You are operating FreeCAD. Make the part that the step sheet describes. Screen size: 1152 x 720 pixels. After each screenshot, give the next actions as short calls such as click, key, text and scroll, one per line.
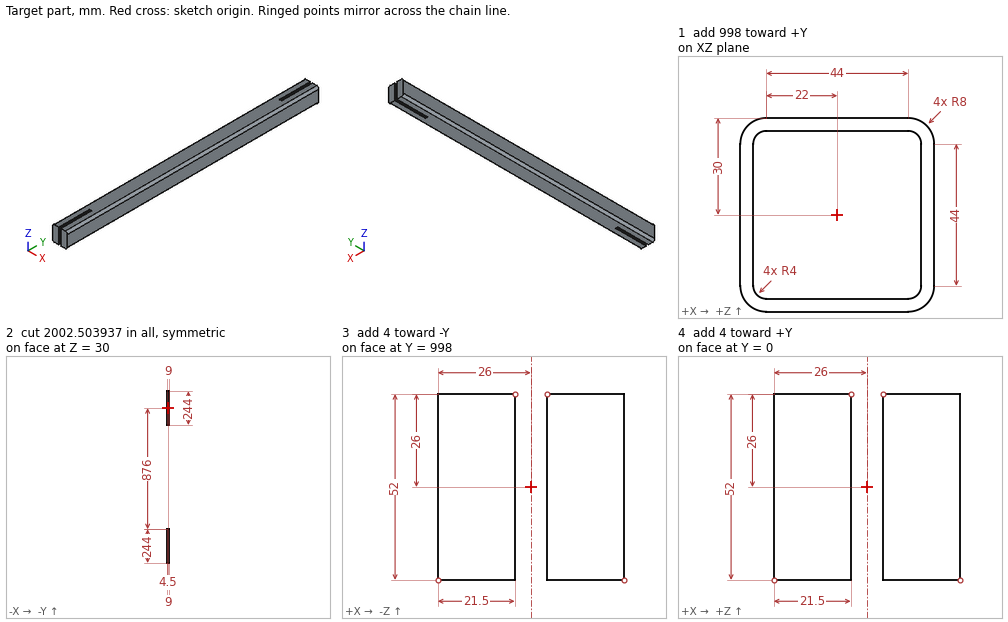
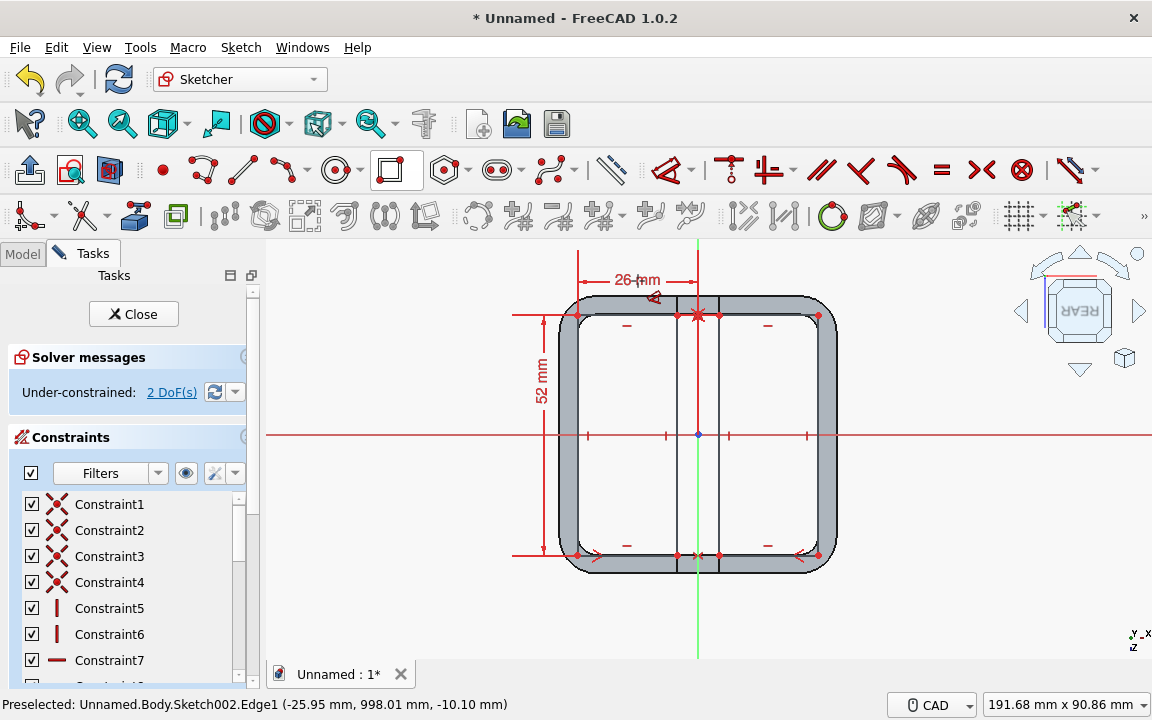
click(578, 315)
click(544, 348)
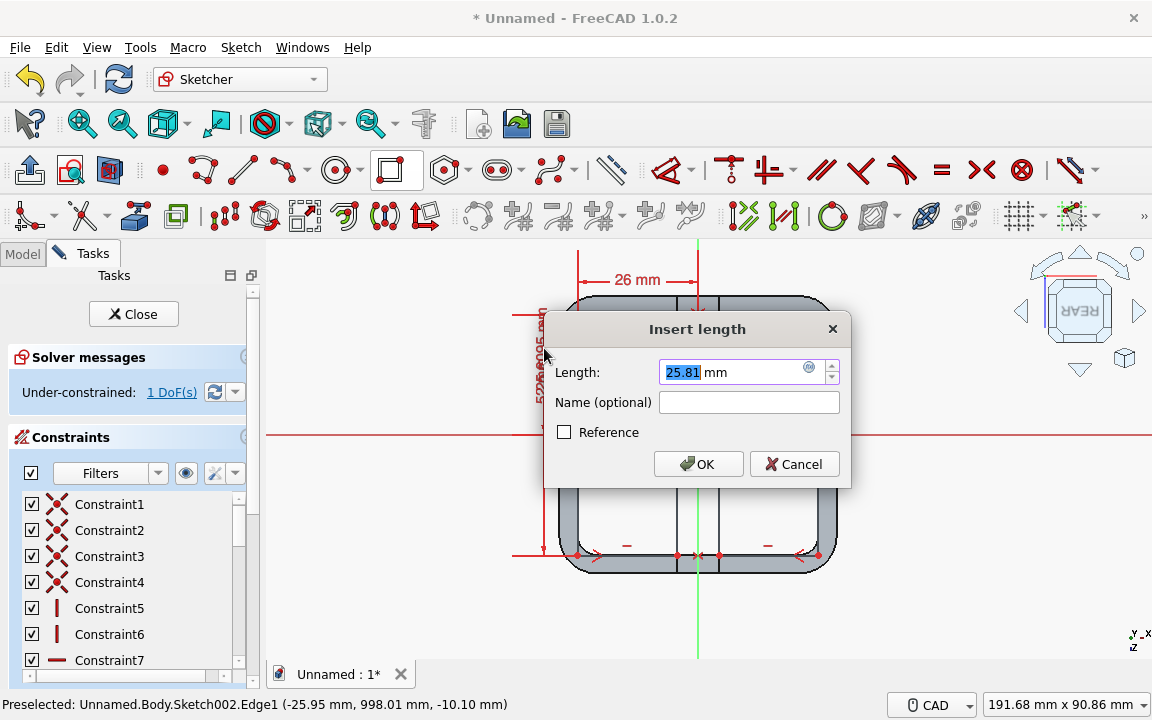
text(26)
key(Return)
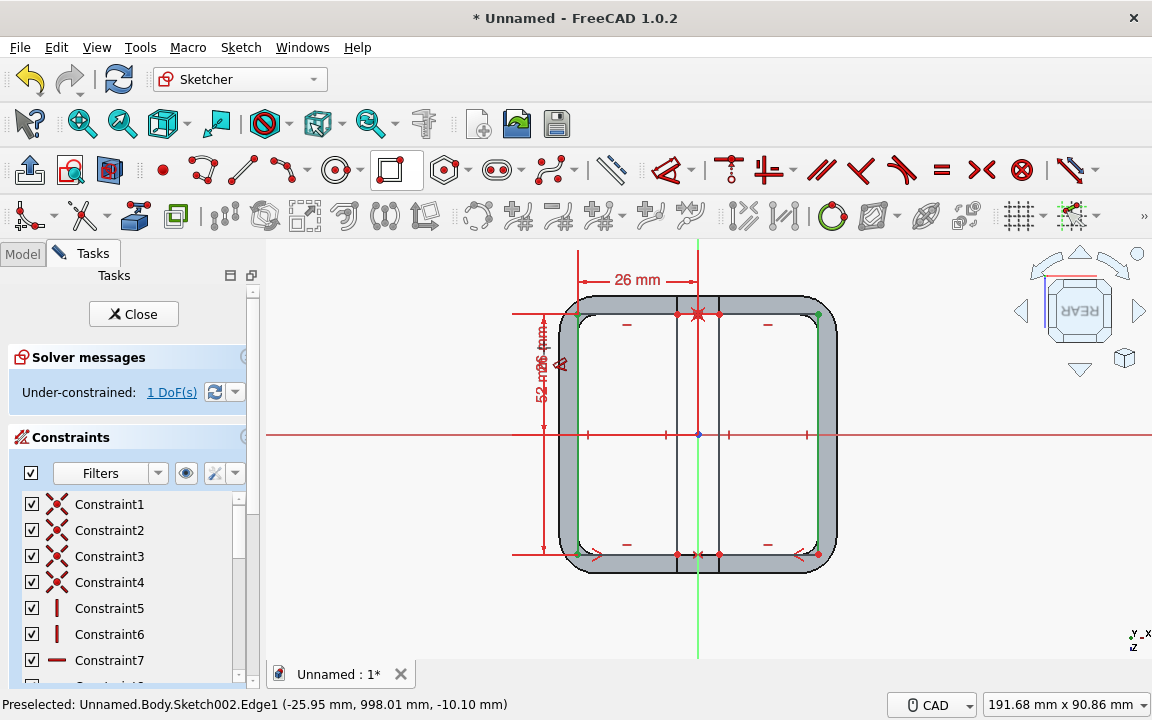
click(608, 555)
click(627, 589)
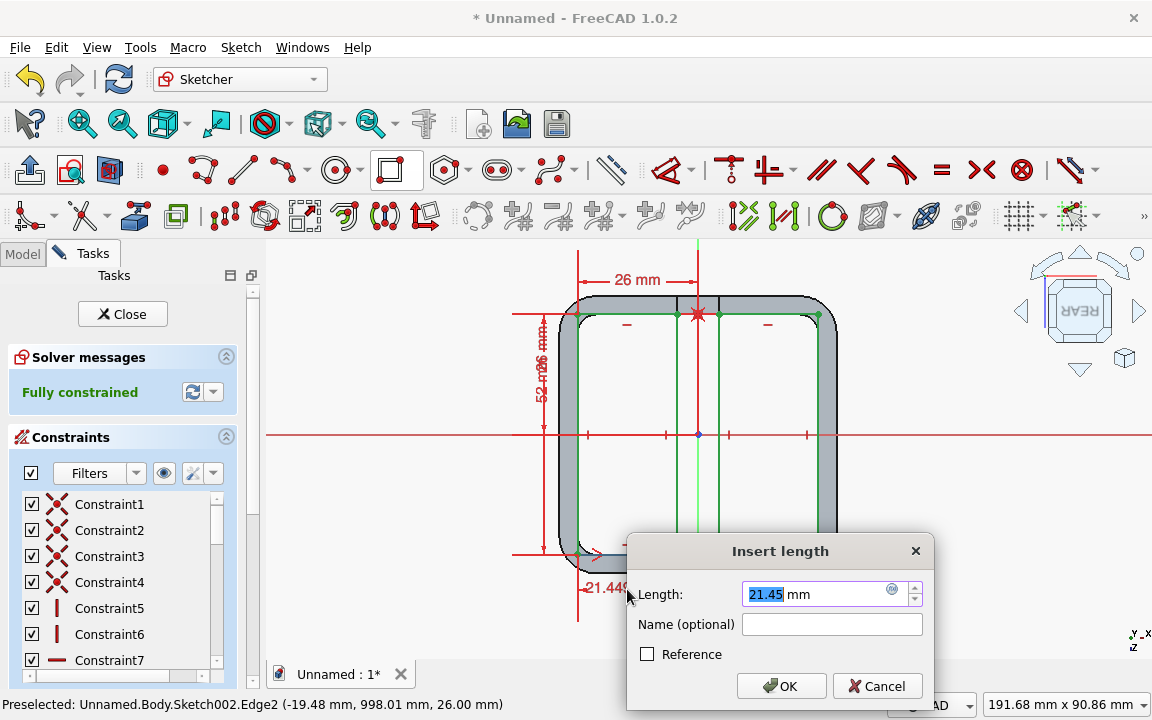
text(21.5)
key(Return)
key(Escape)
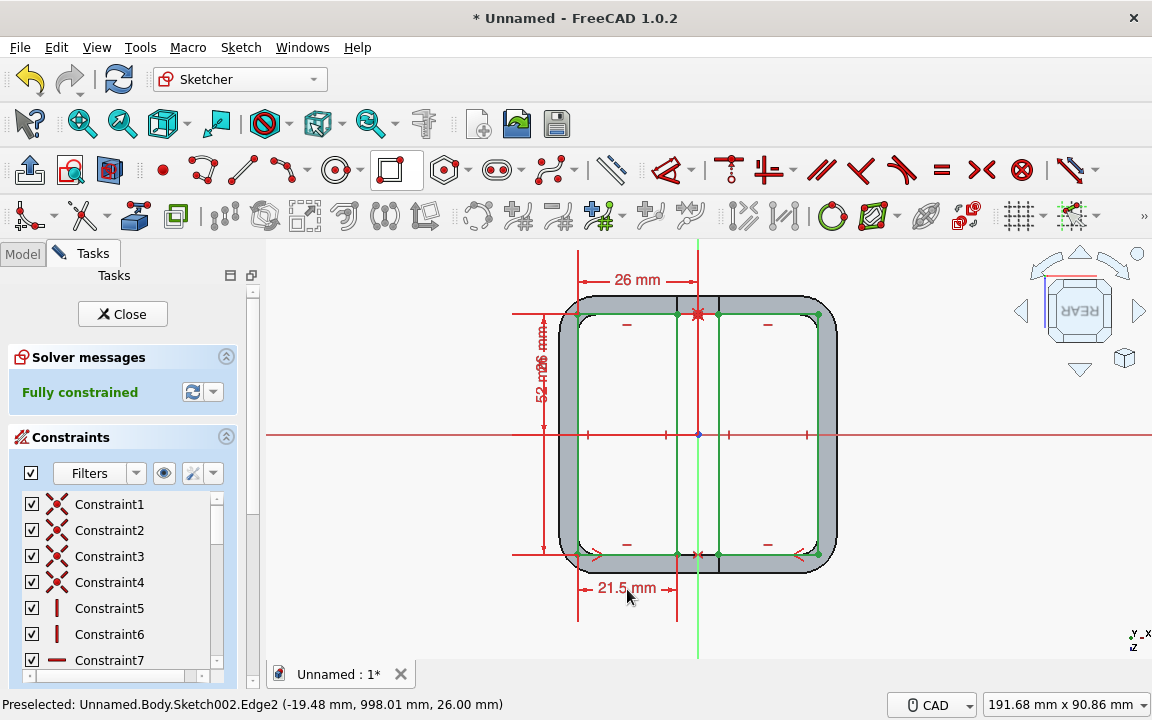
click(123, 314)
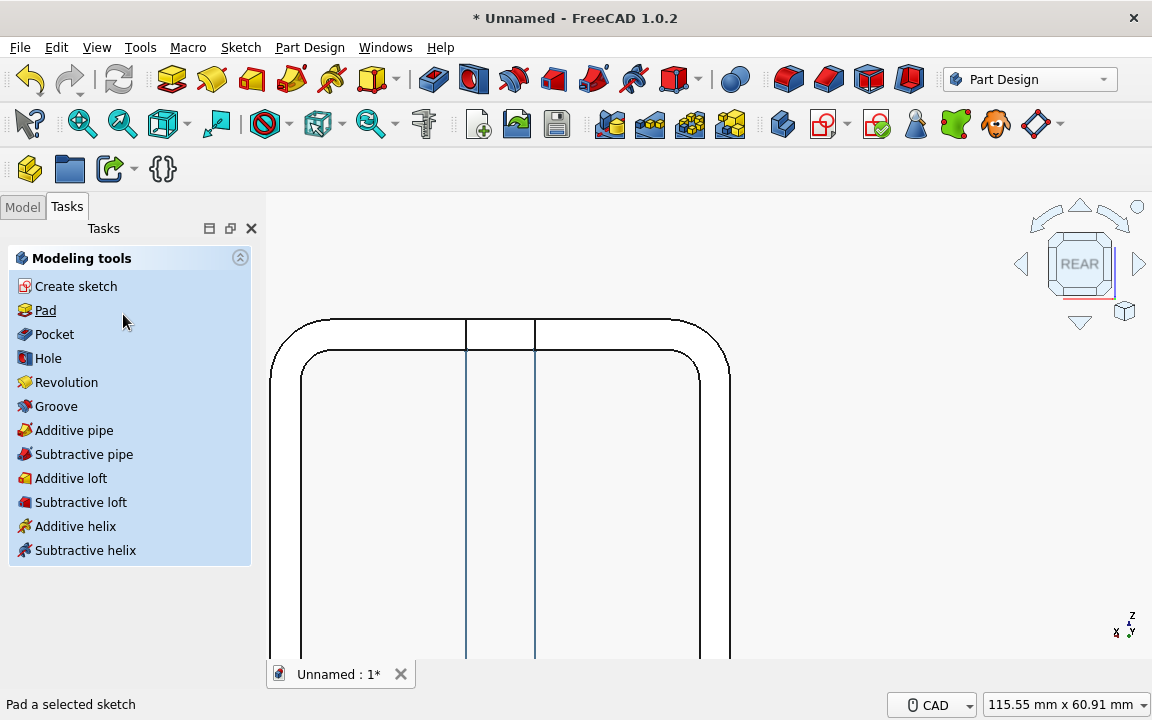
click(172, 80)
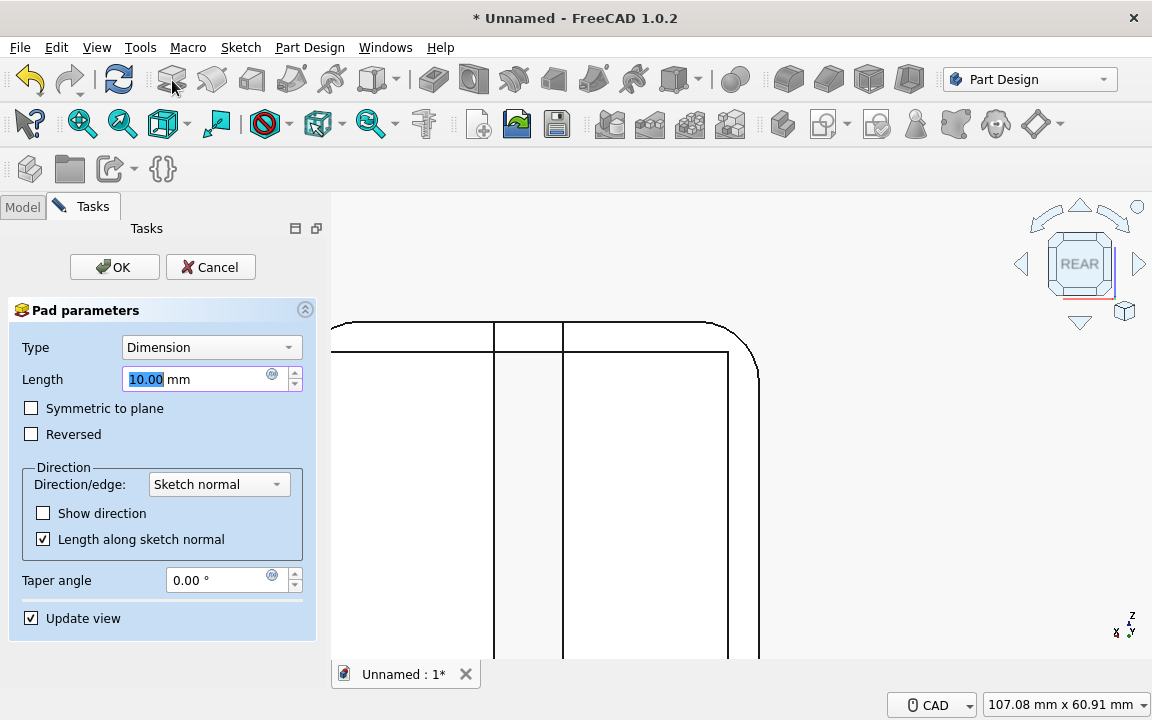
text(4)
key(Tab)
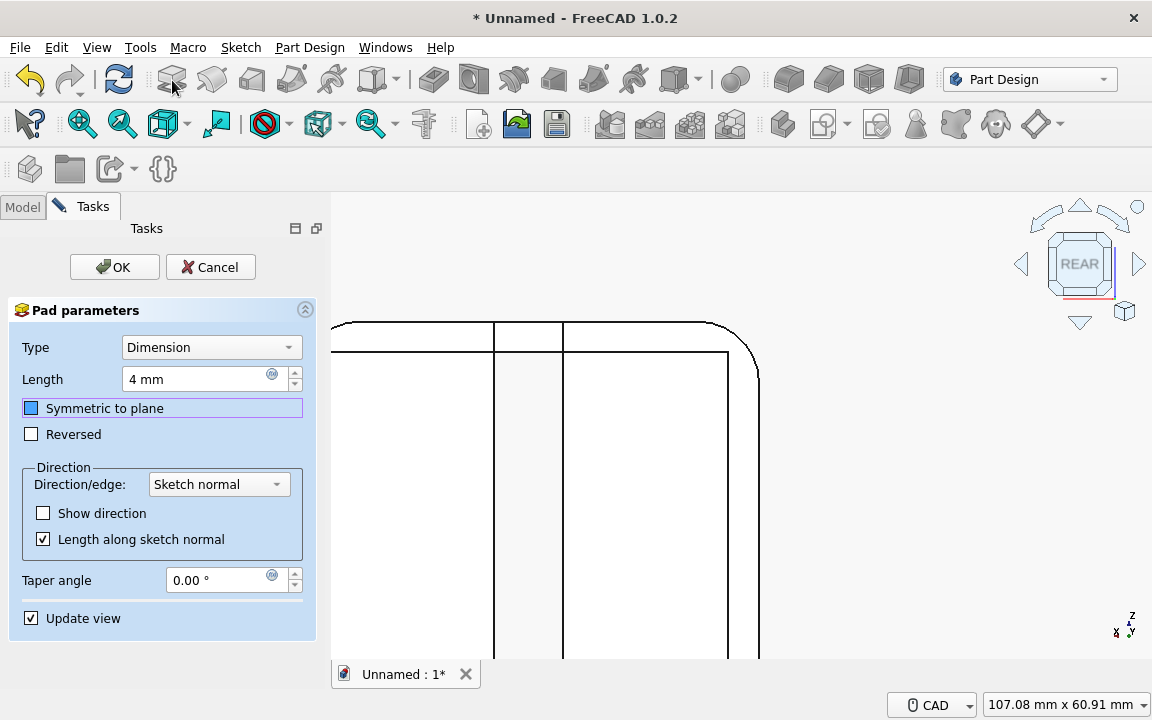
click(30, 434)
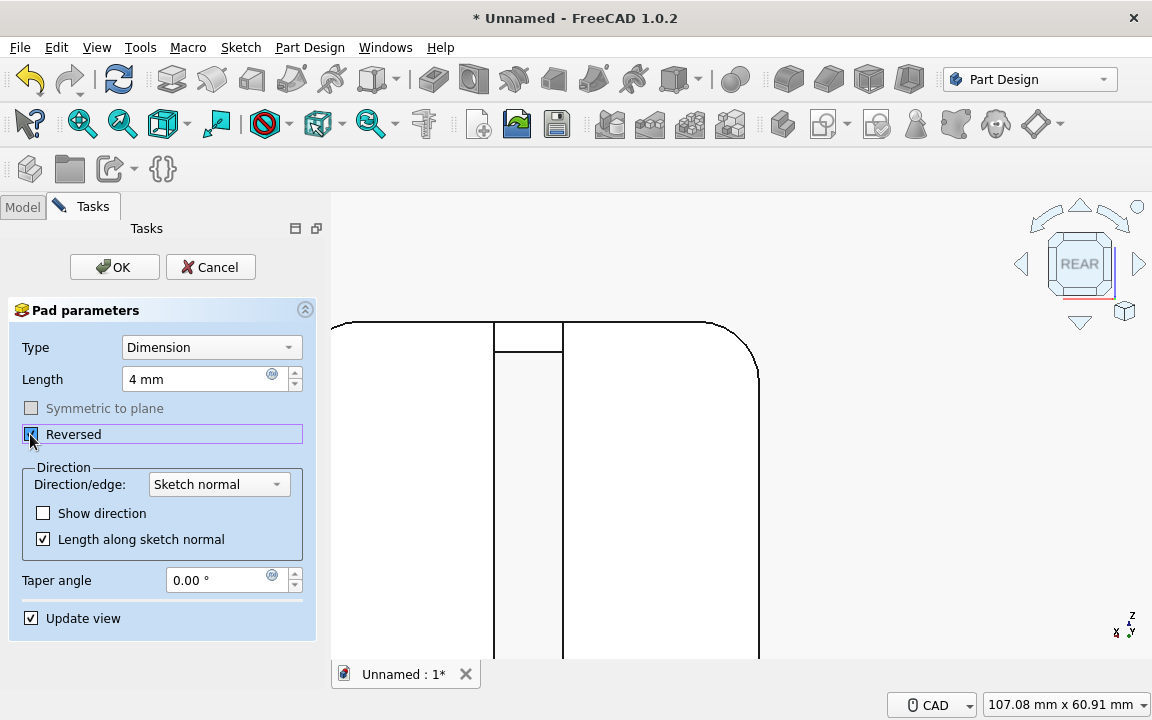
click(115, 267)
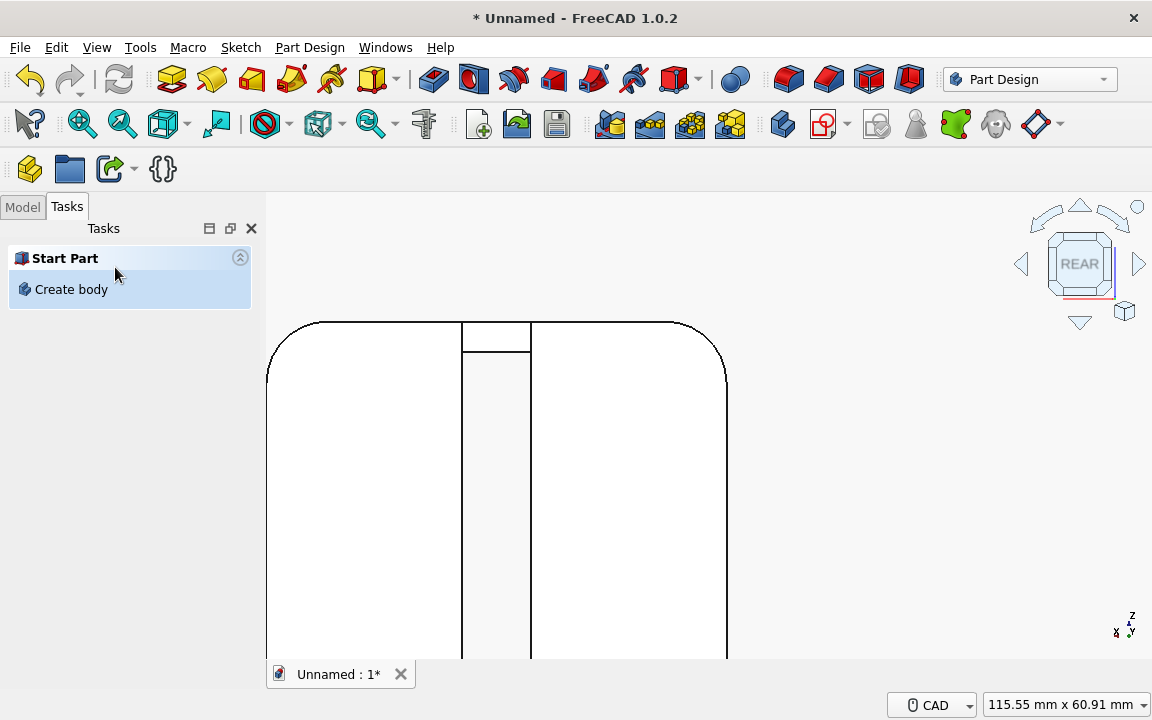
click(84, 124)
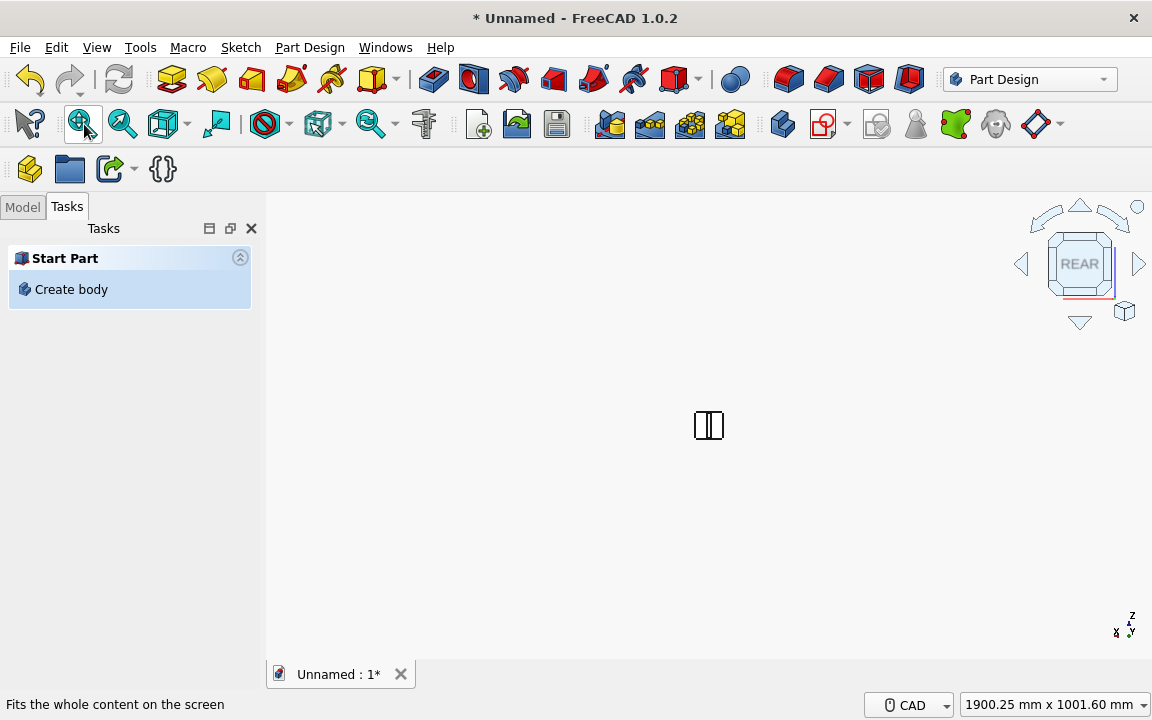
key(0)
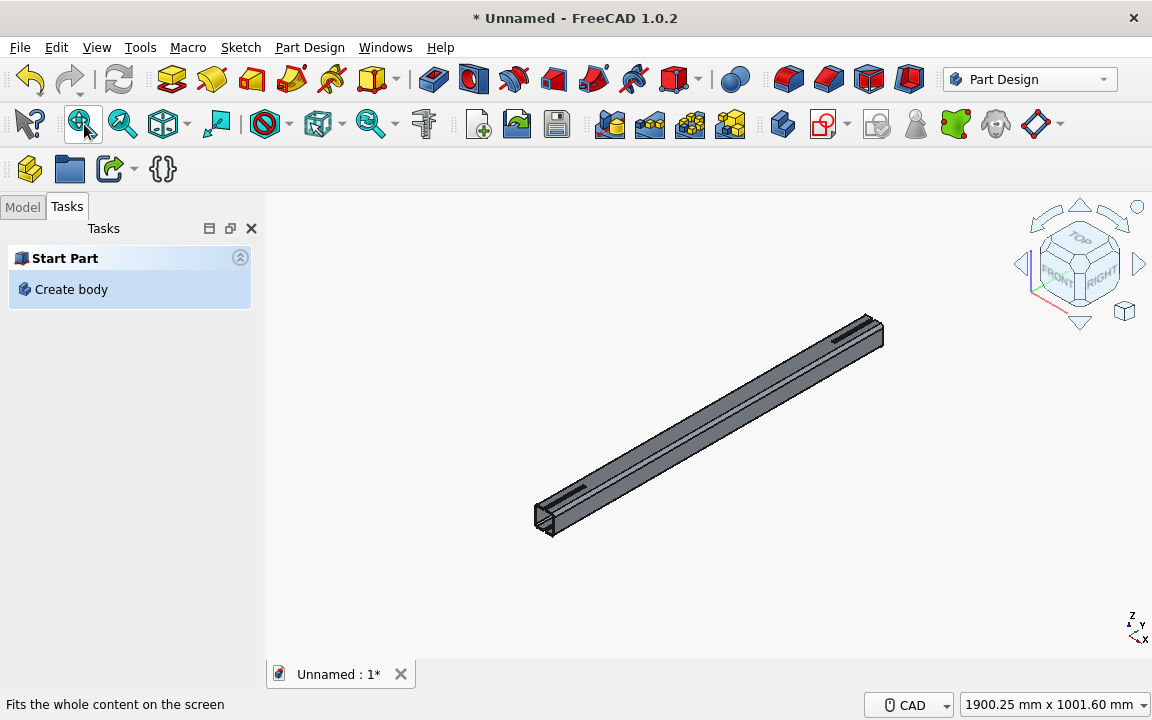
scroll(535, 508, up, 14)